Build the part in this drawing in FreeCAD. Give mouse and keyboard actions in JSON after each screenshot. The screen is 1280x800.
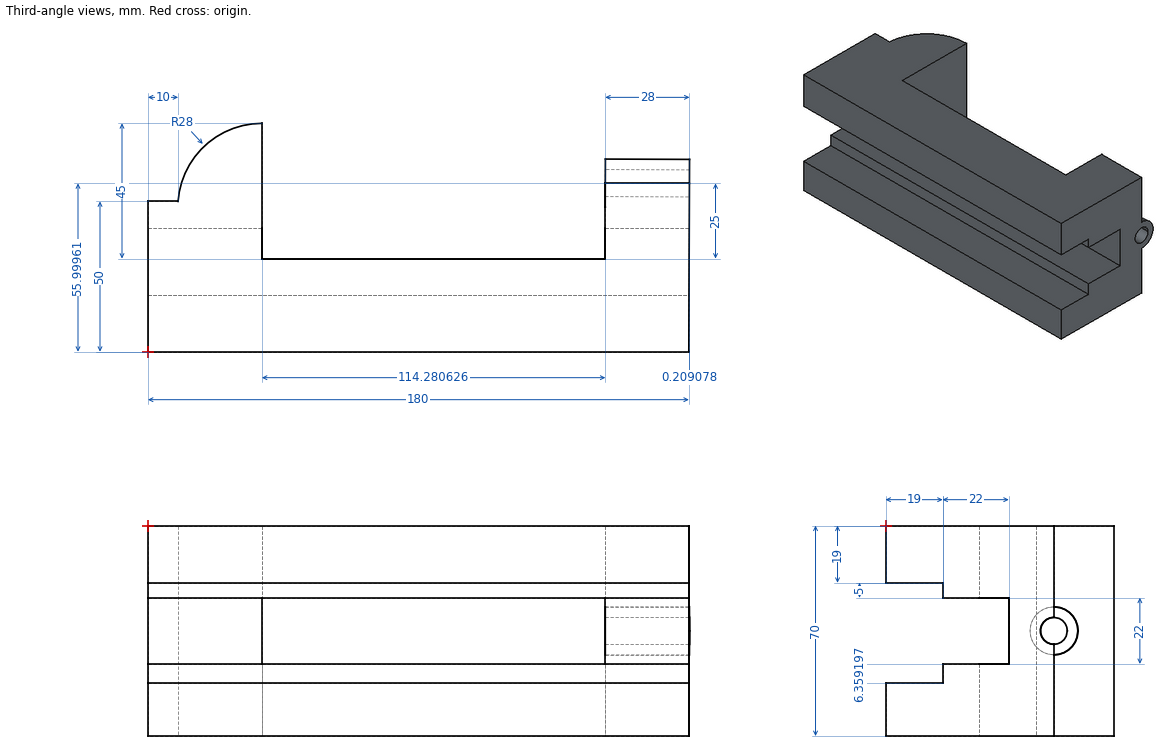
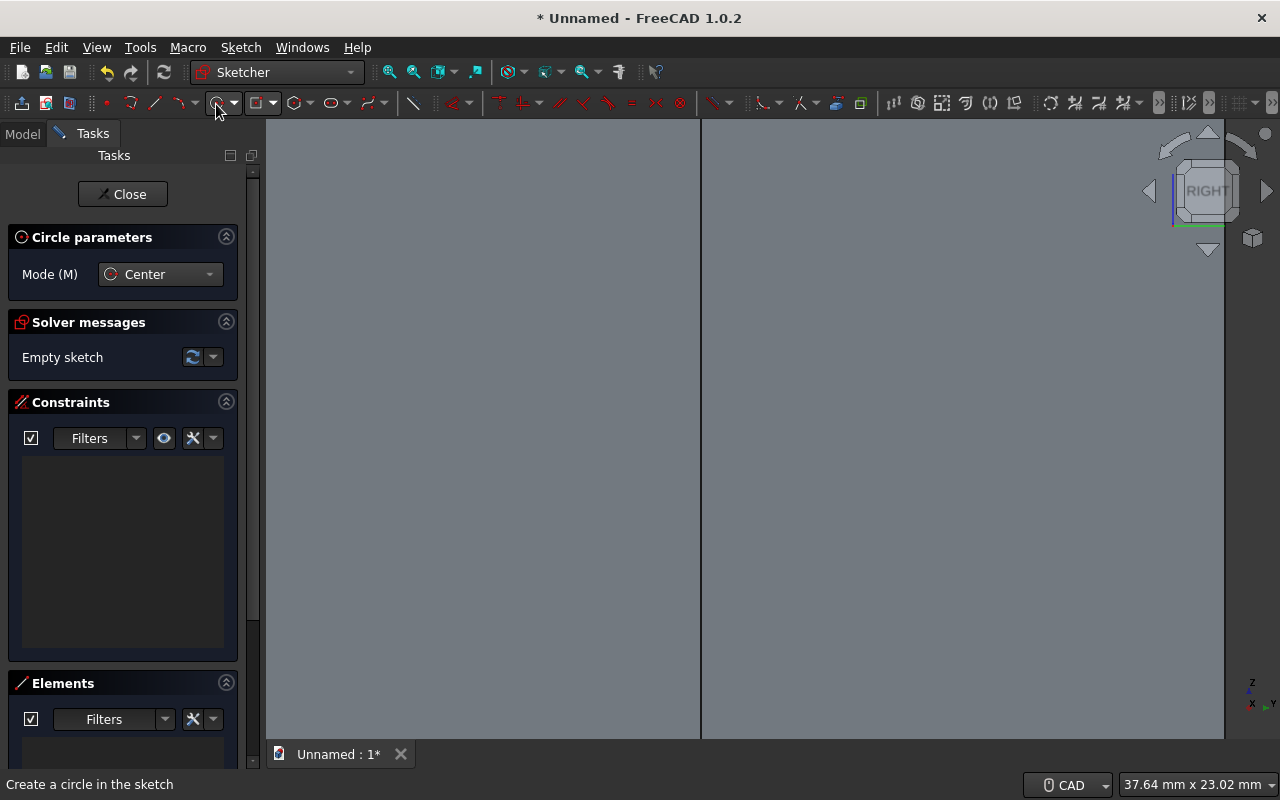
{"action": "left_click", "coordinate": [701, 425]}
{"action": "mouse_move", "coordinate": [853, 273]}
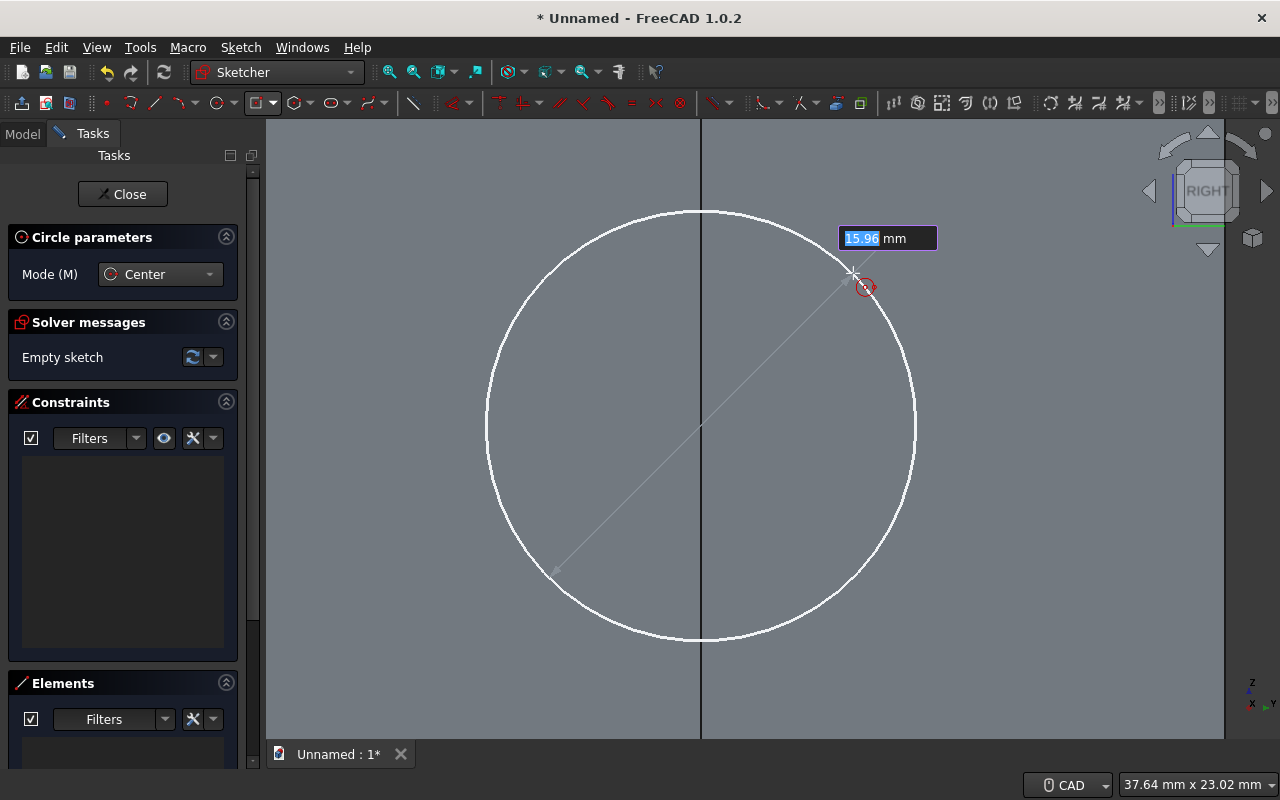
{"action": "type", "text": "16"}
{"action": "key", "text": "Return"}
{"action": "key", "text": "Escape"}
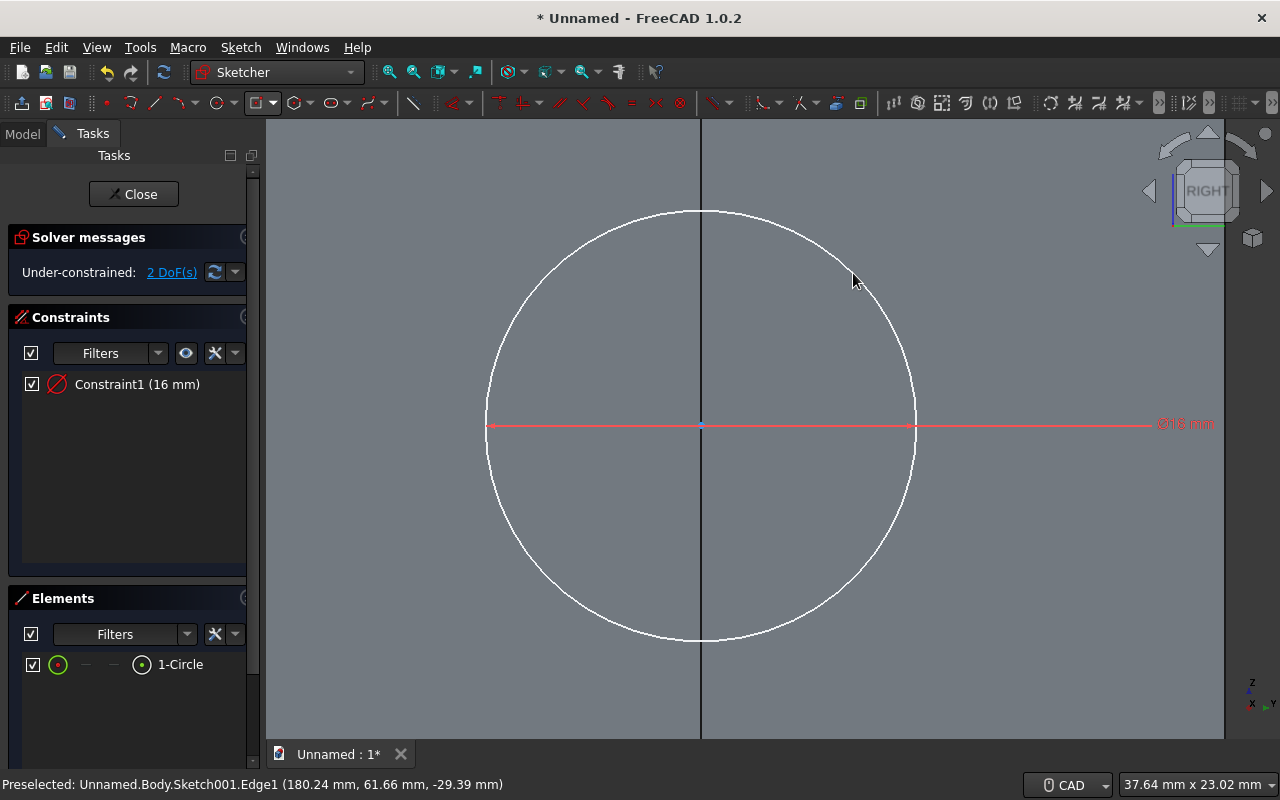
{"action": "left_click", "coordinate": [701, 426]}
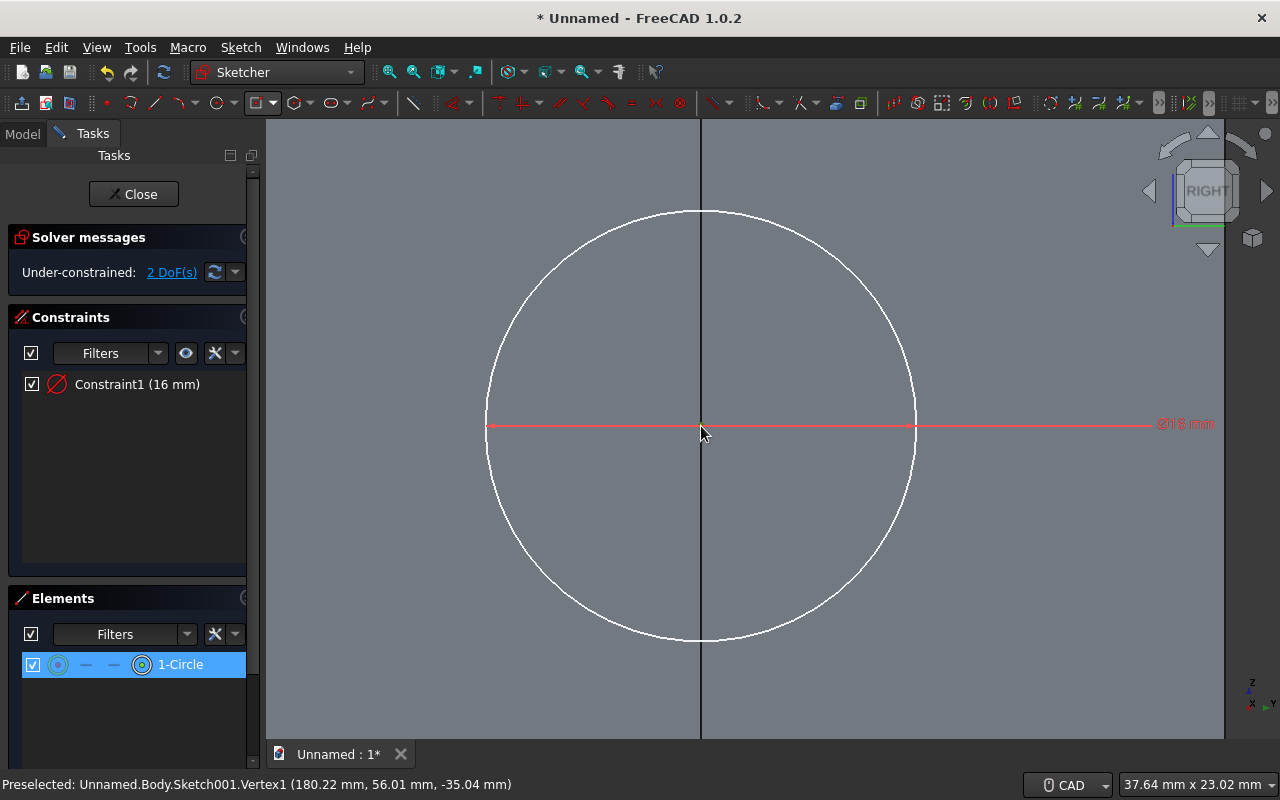
{"action": "key", "text": "i"}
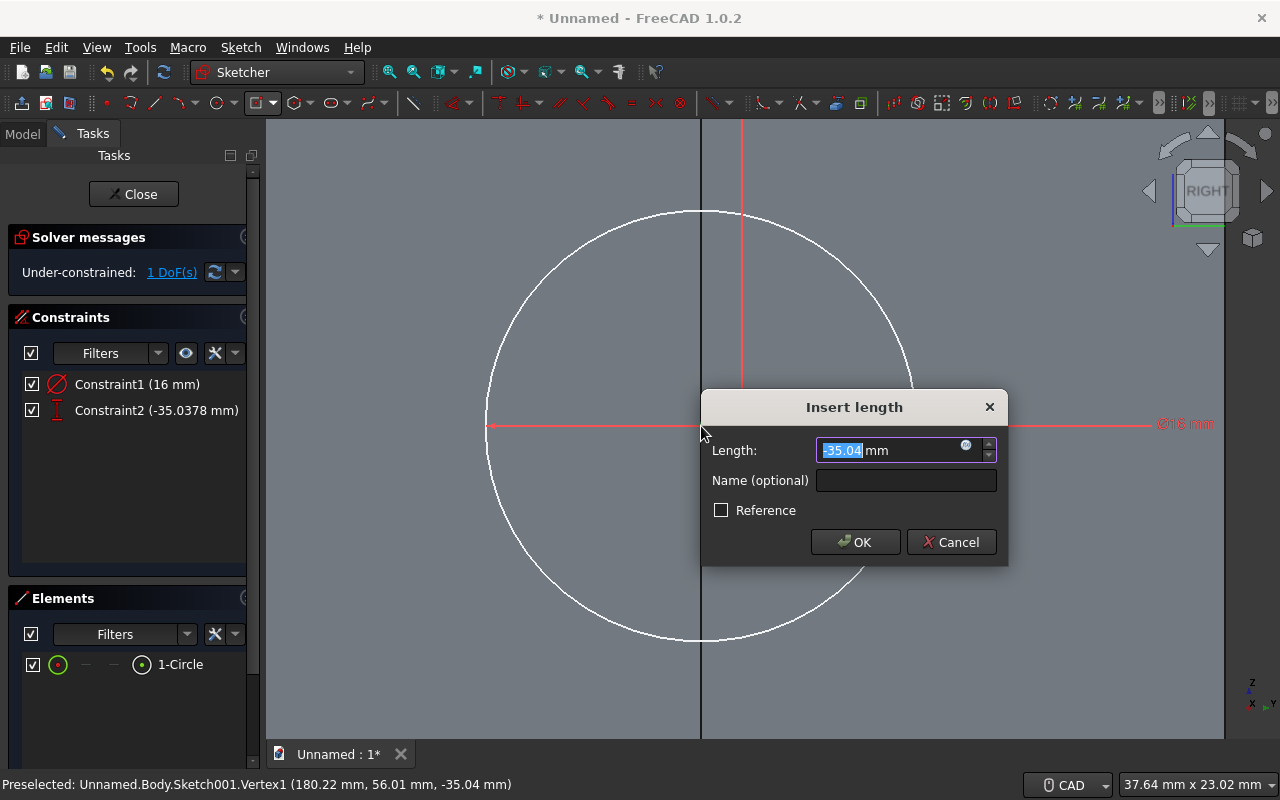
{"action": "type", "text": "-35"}
{"action": "key", "text": "Return"}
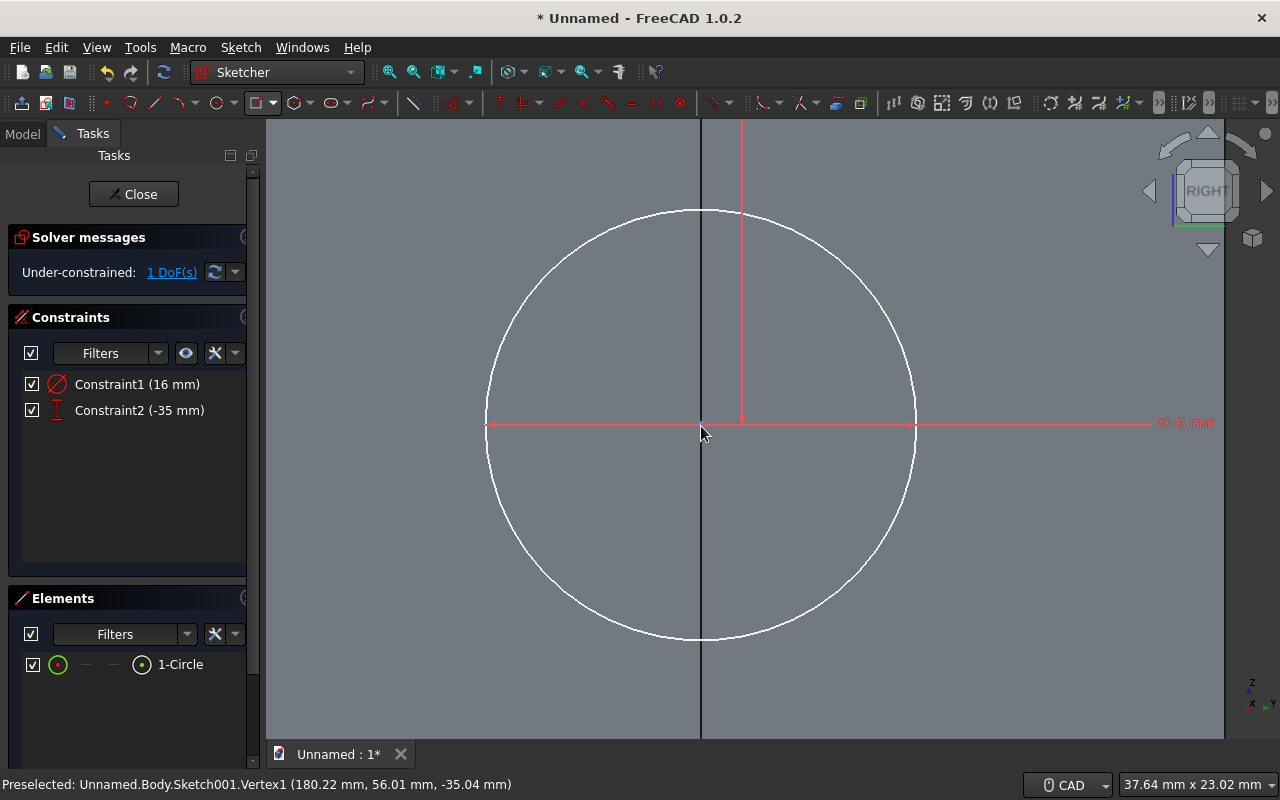
{"action": "left_click", "coordinate": [701, 425]}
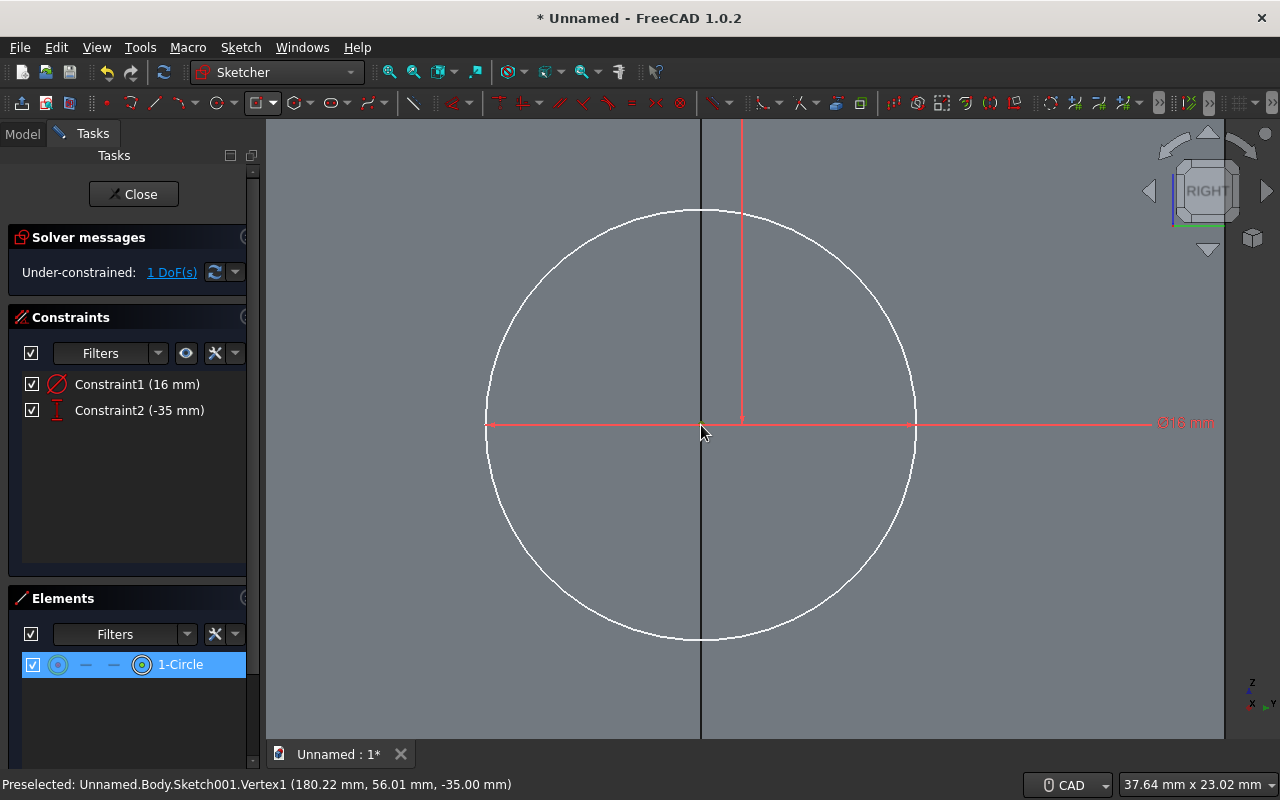
{"action": "left_click", "coordinate": [472, 104]}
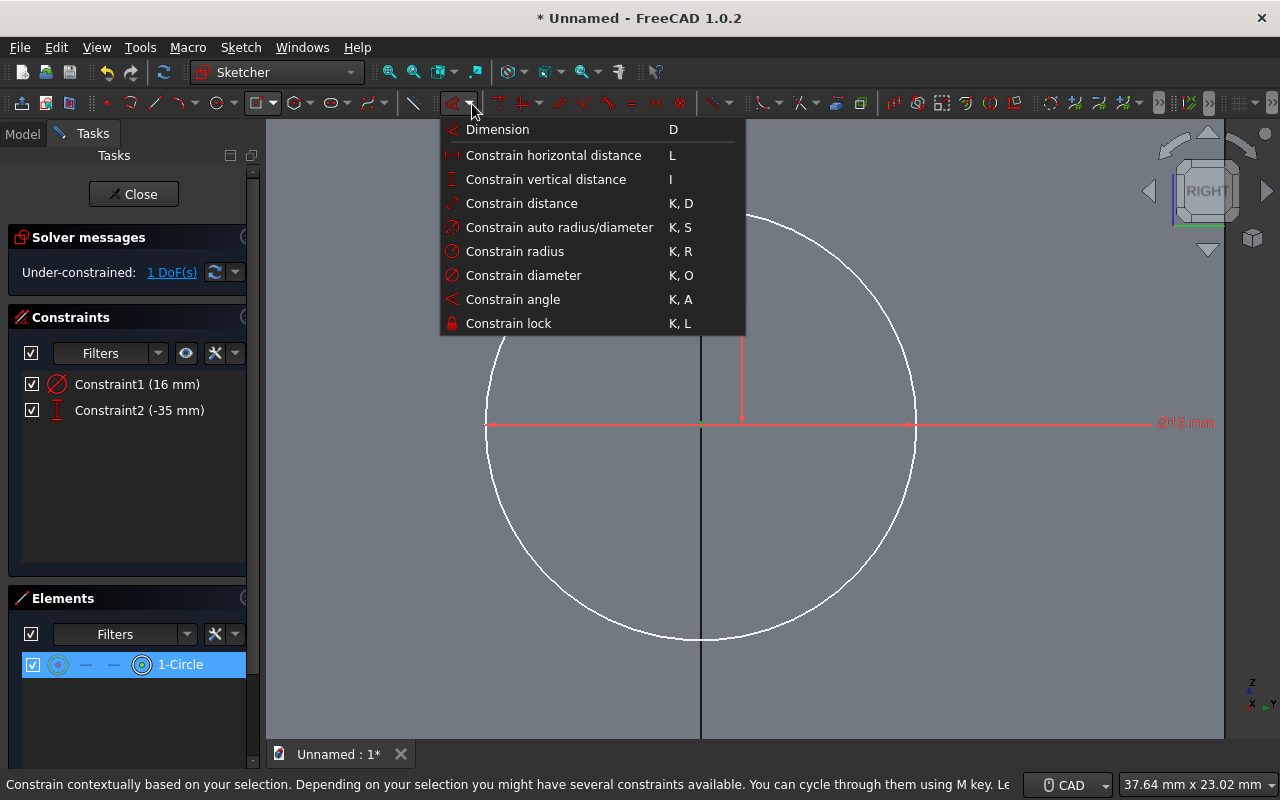
{"action": "left_click", "coordinate": [593, 155]}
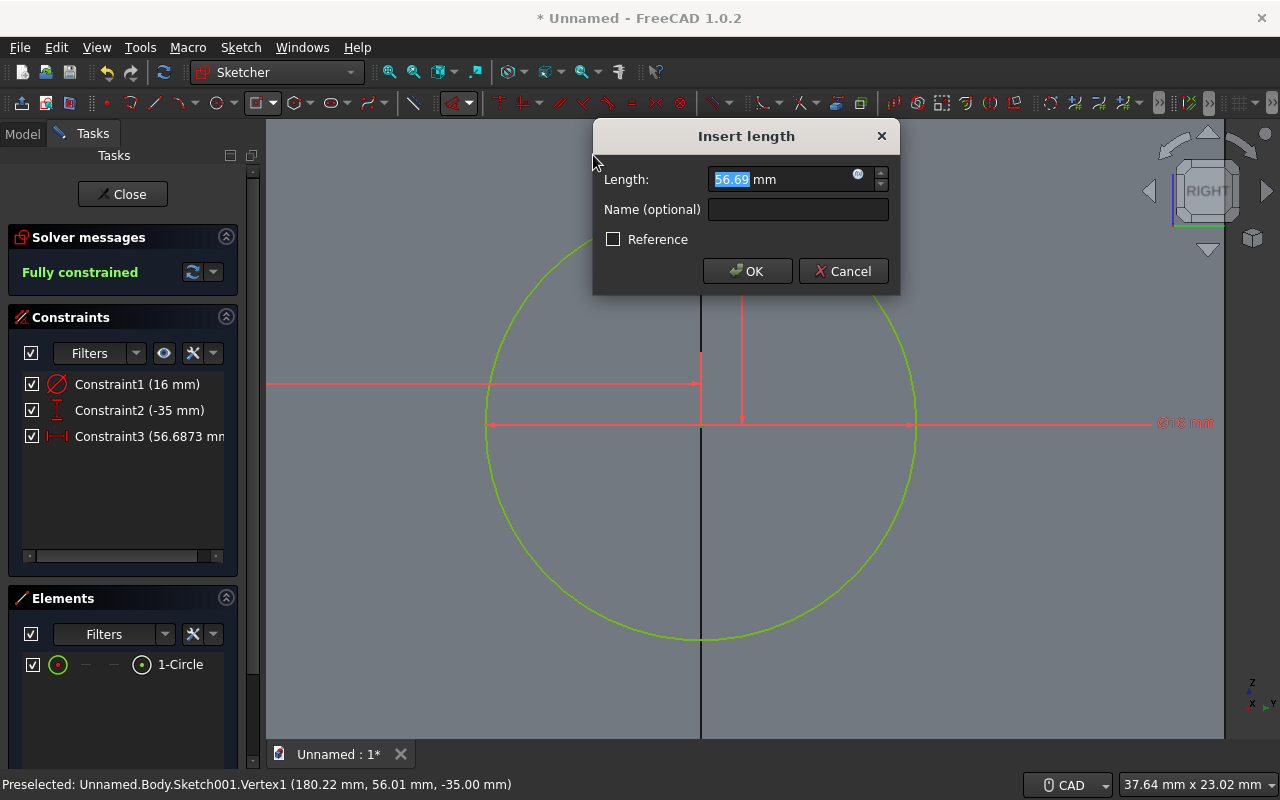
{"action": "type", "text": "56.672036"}
{"action": "key", "text": "Return"}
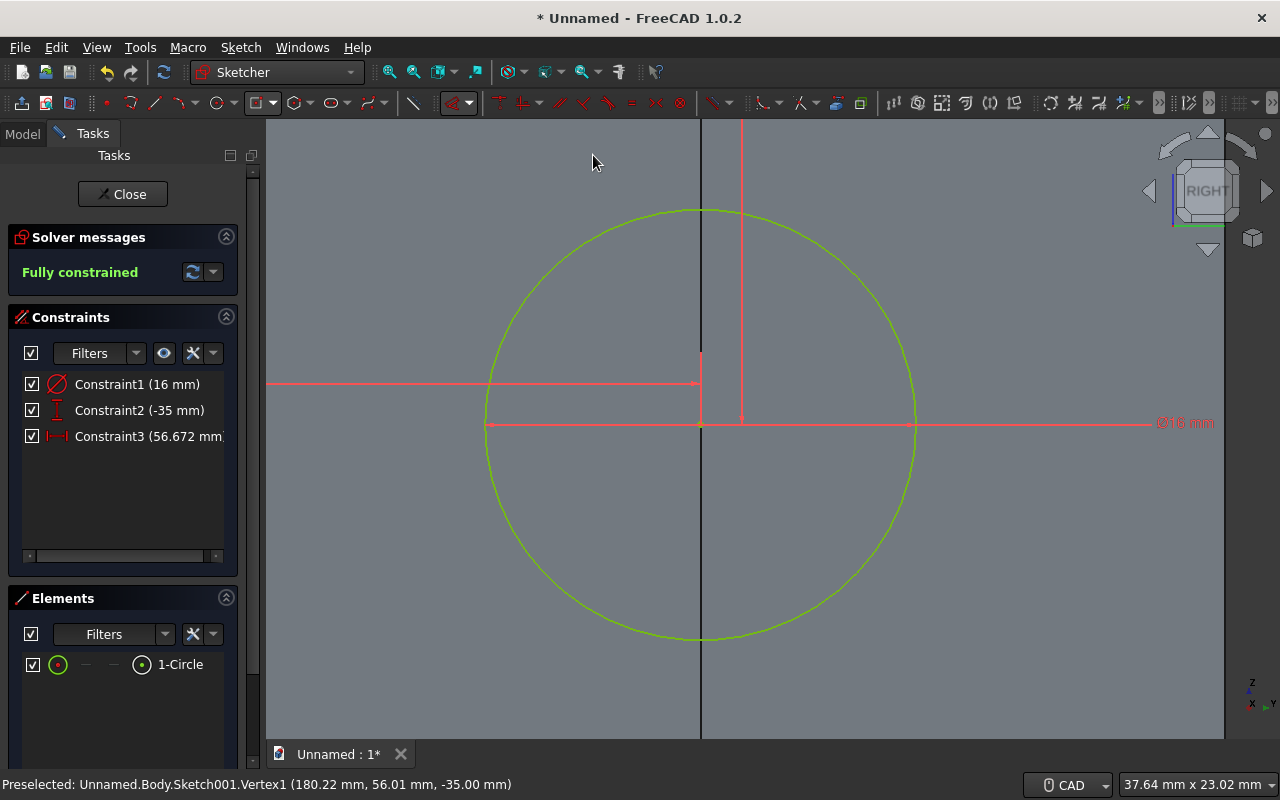
{"action": "left_click", "coordinate": [123, 194]}